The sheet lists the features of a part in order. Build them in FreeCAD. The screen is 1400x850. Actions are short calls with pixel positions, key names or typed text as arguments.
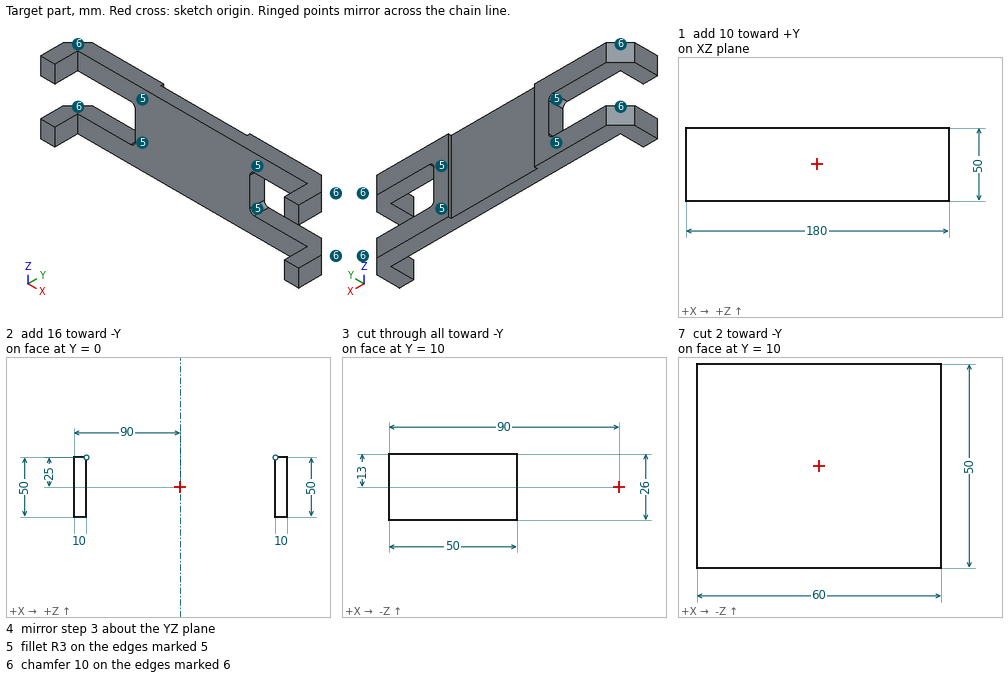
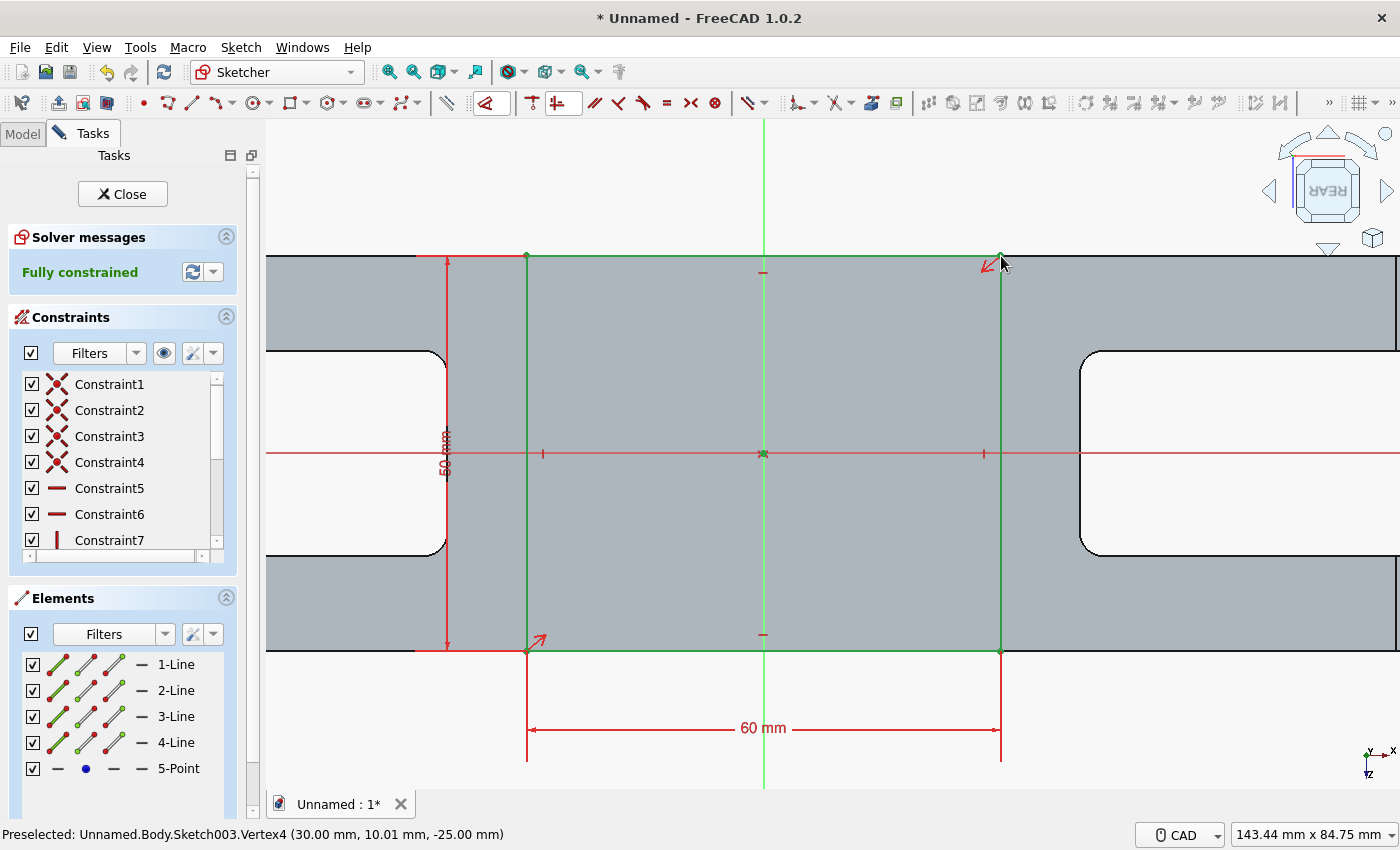
click(123, 194)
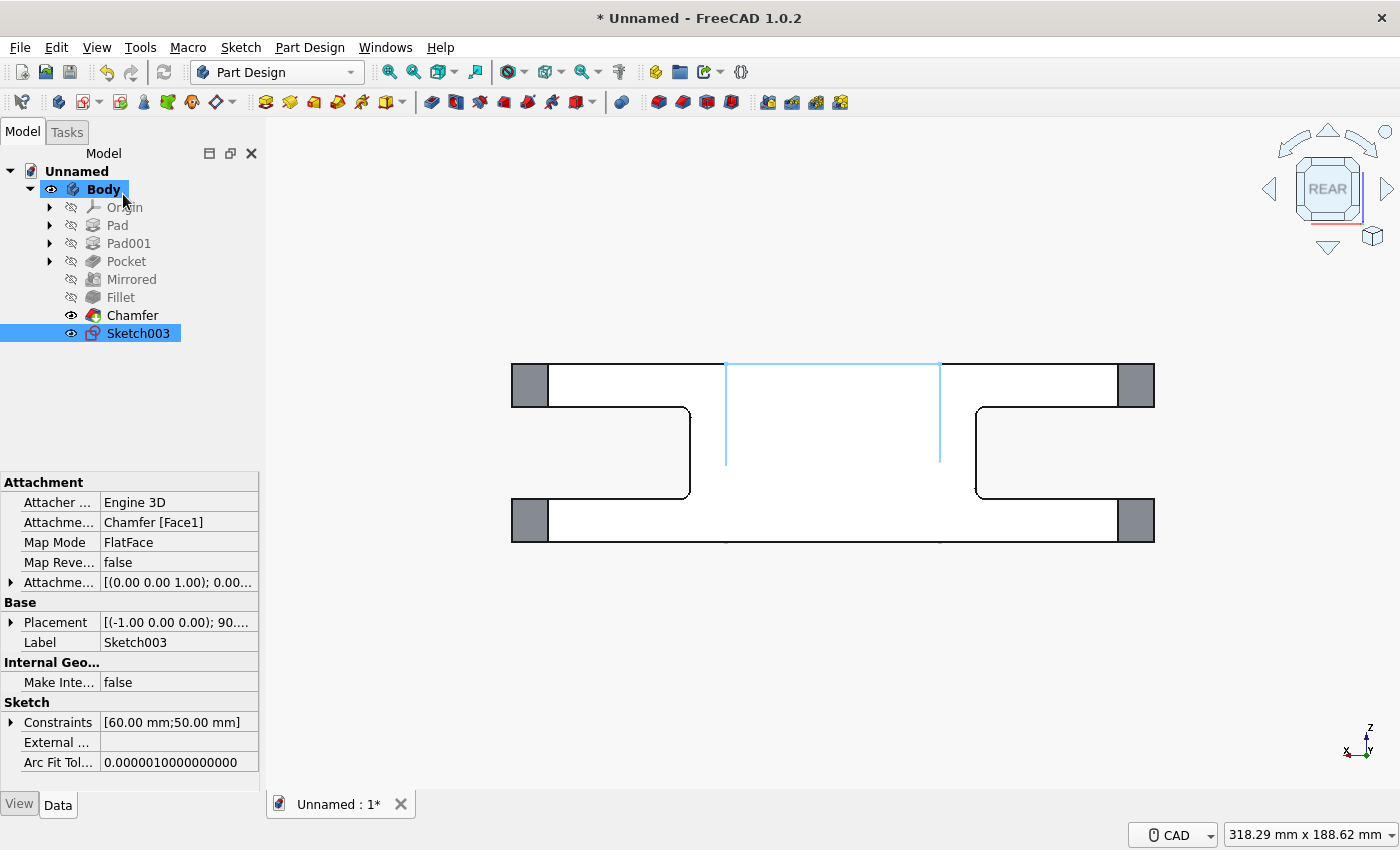
click(432, 102)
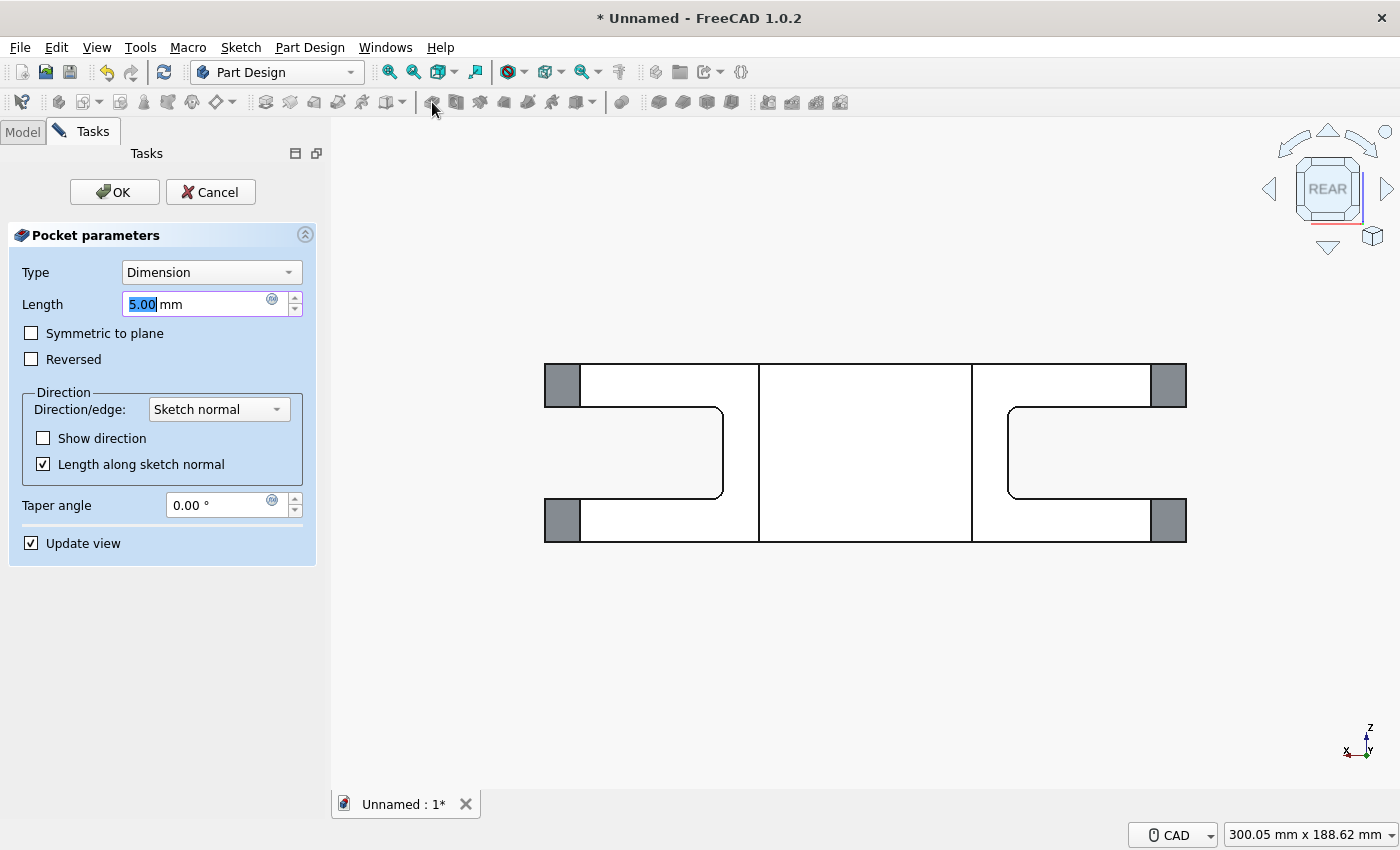
text(2)
key(Tab)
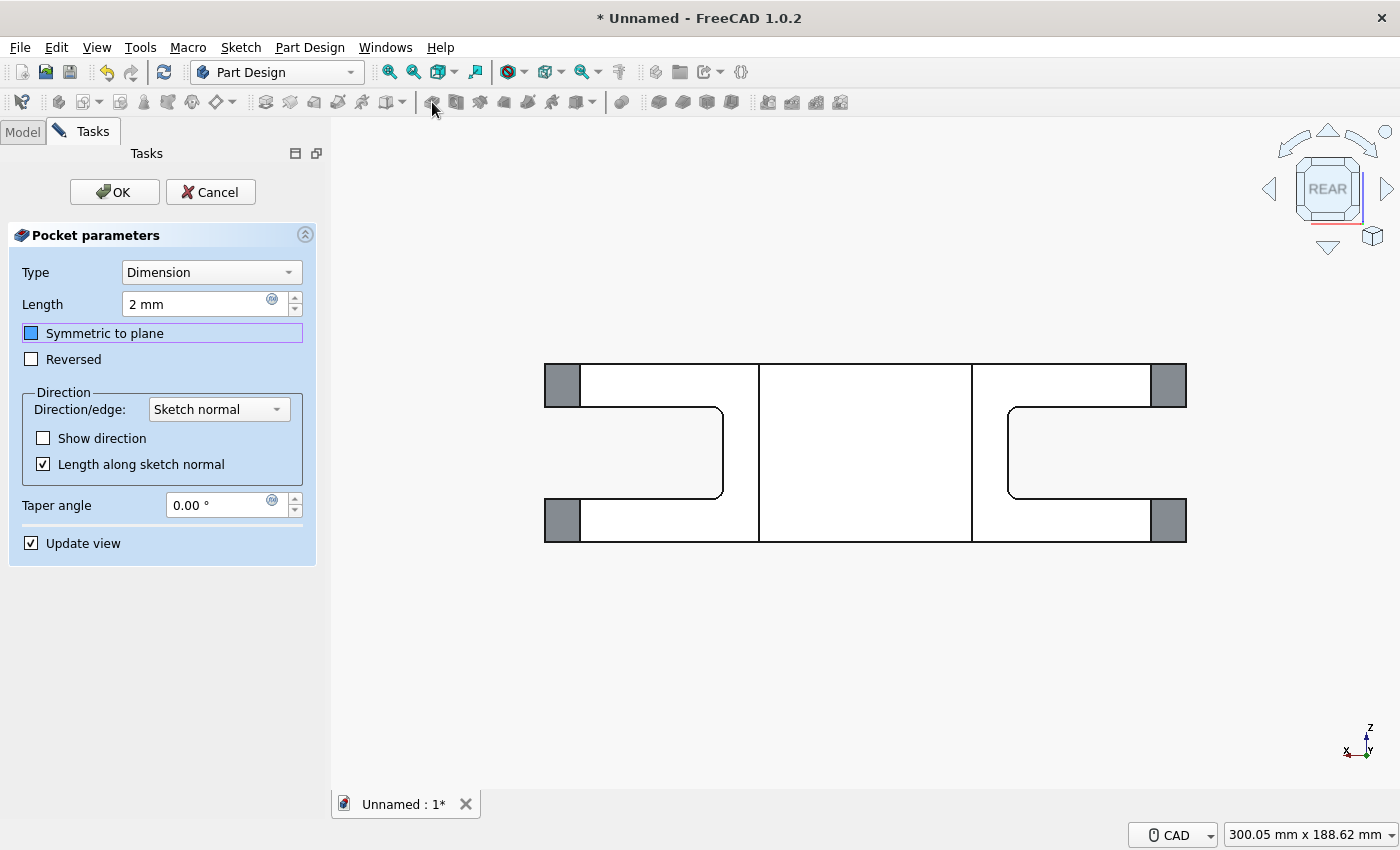
click(115, 192)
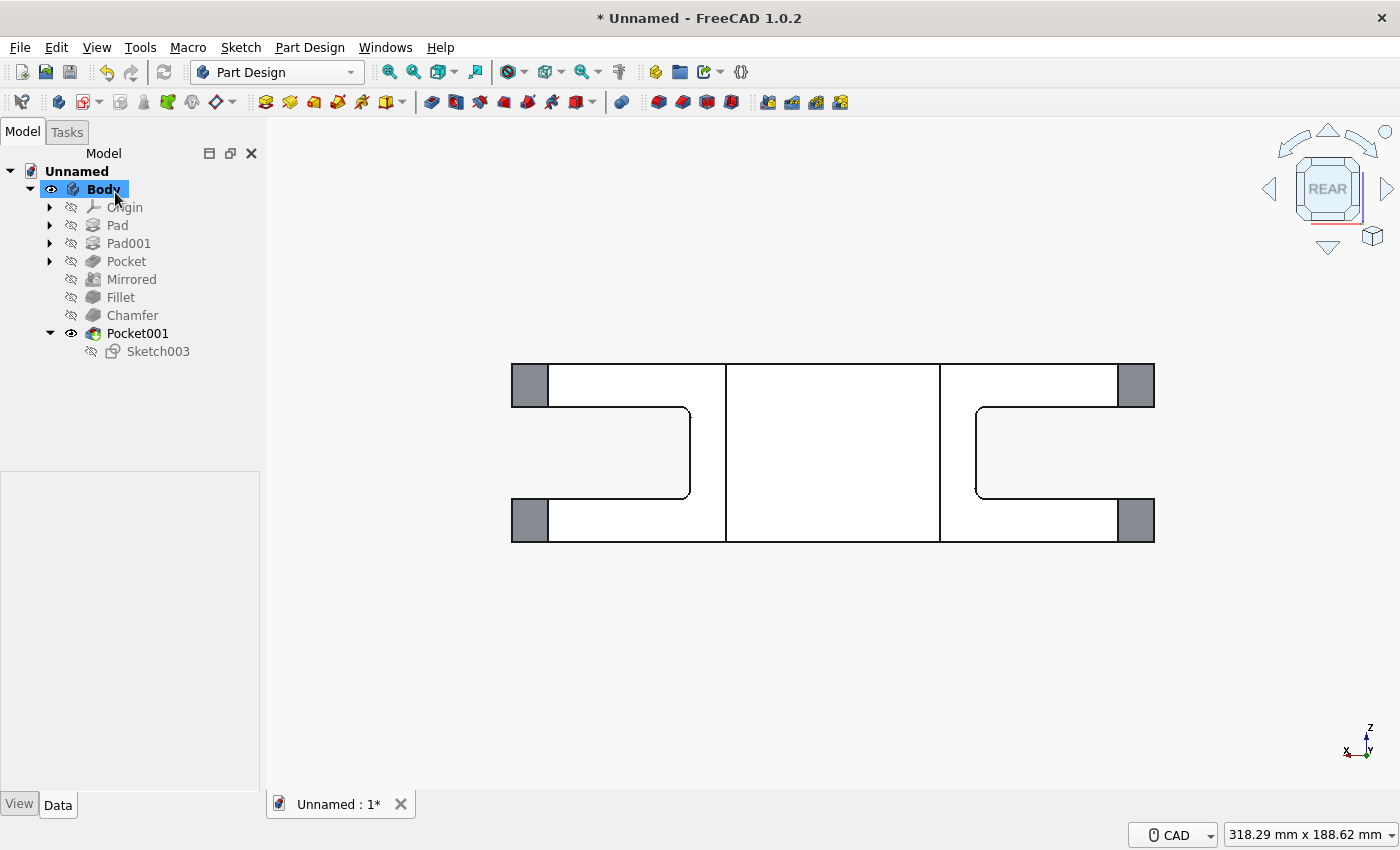
key(0)